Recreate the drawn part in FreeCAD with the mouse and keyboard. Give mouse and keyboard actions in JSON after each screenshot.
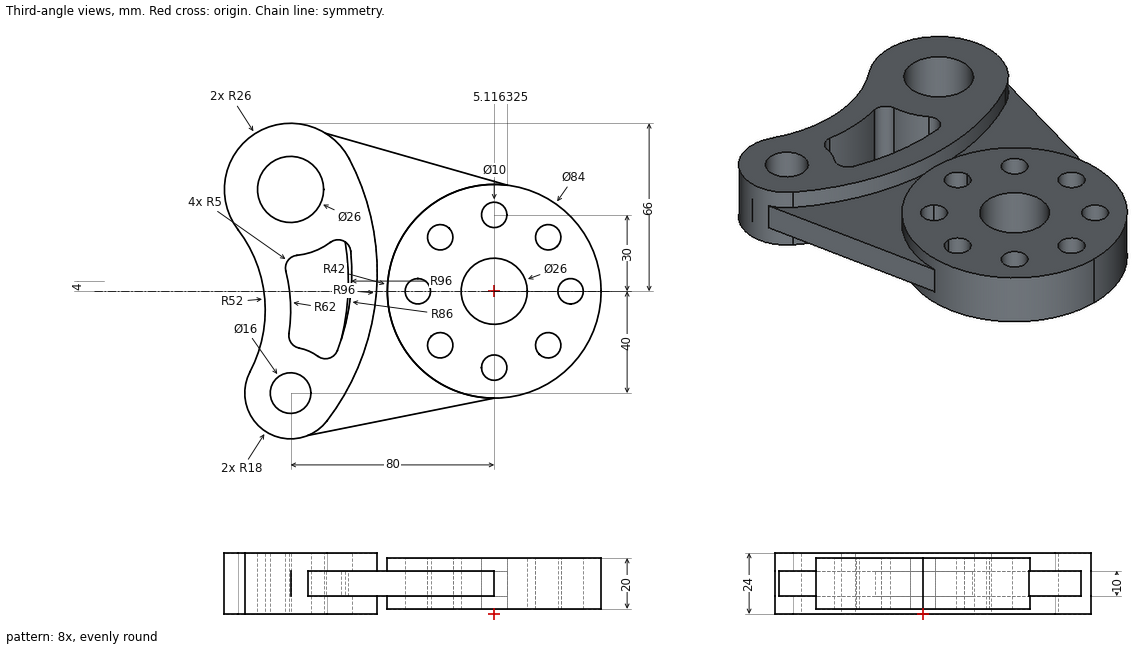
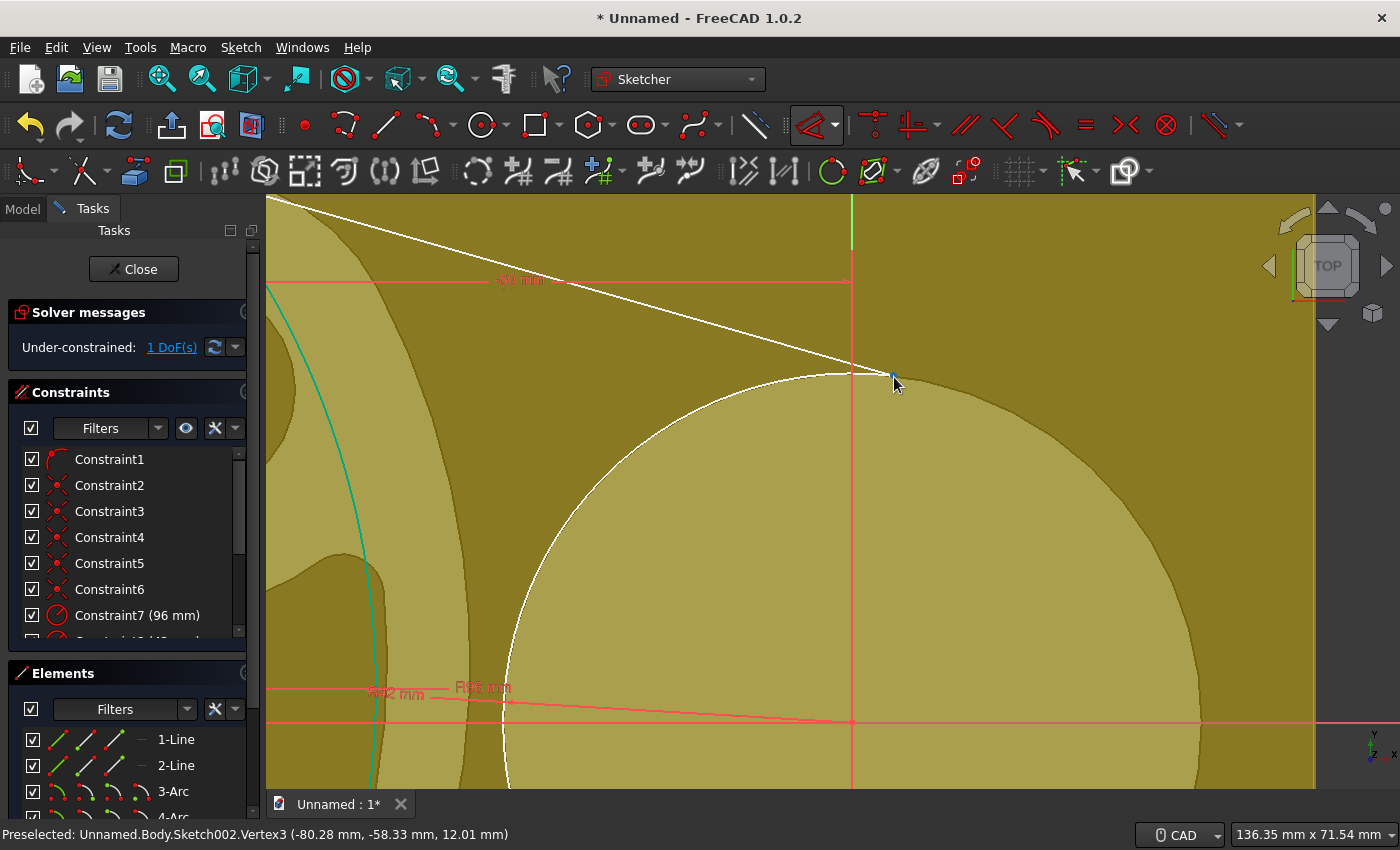
{"action": "left_click", "coordinate": [894, 376]}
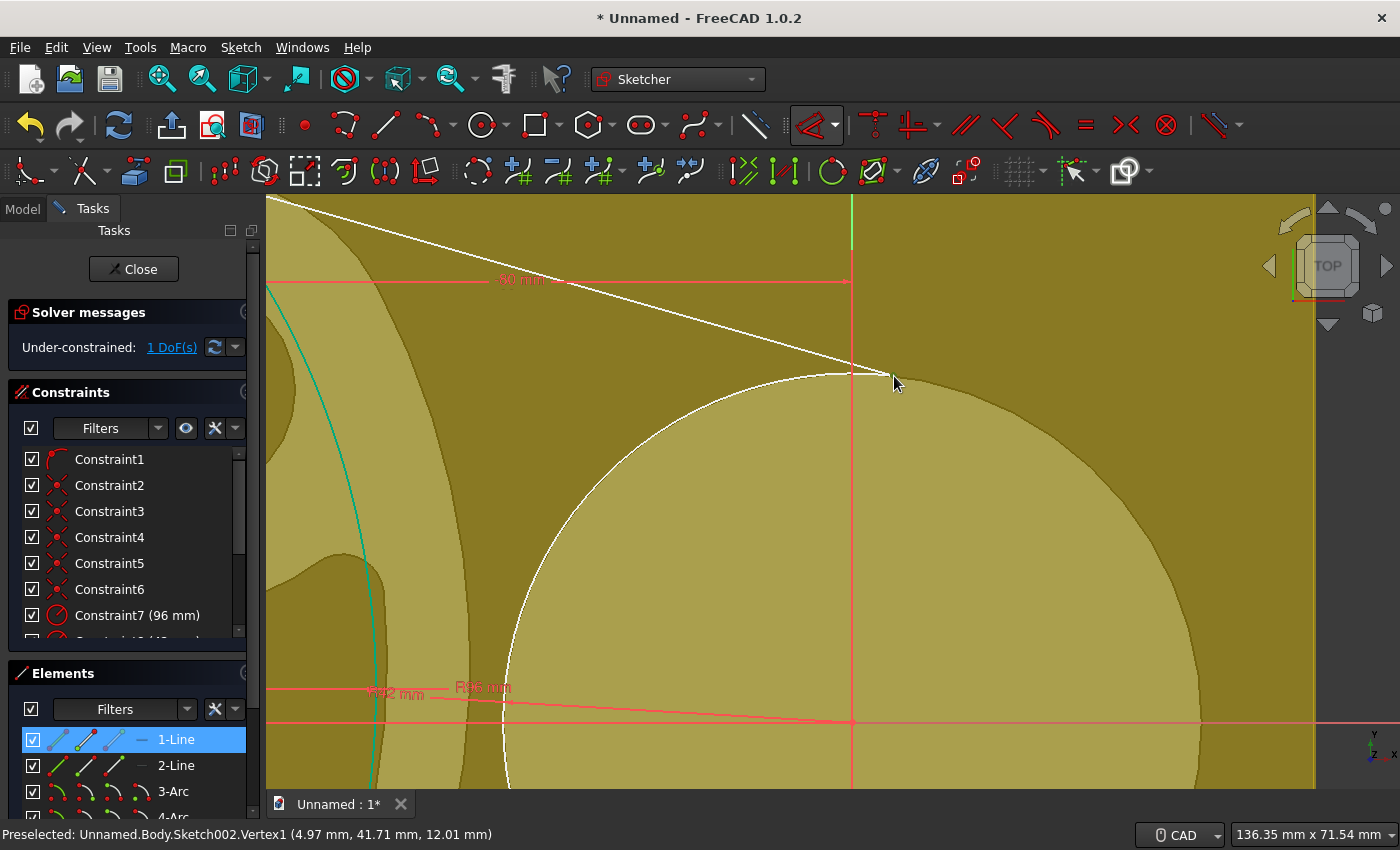
{"action": "left_click", "coordinate": [838, 126]}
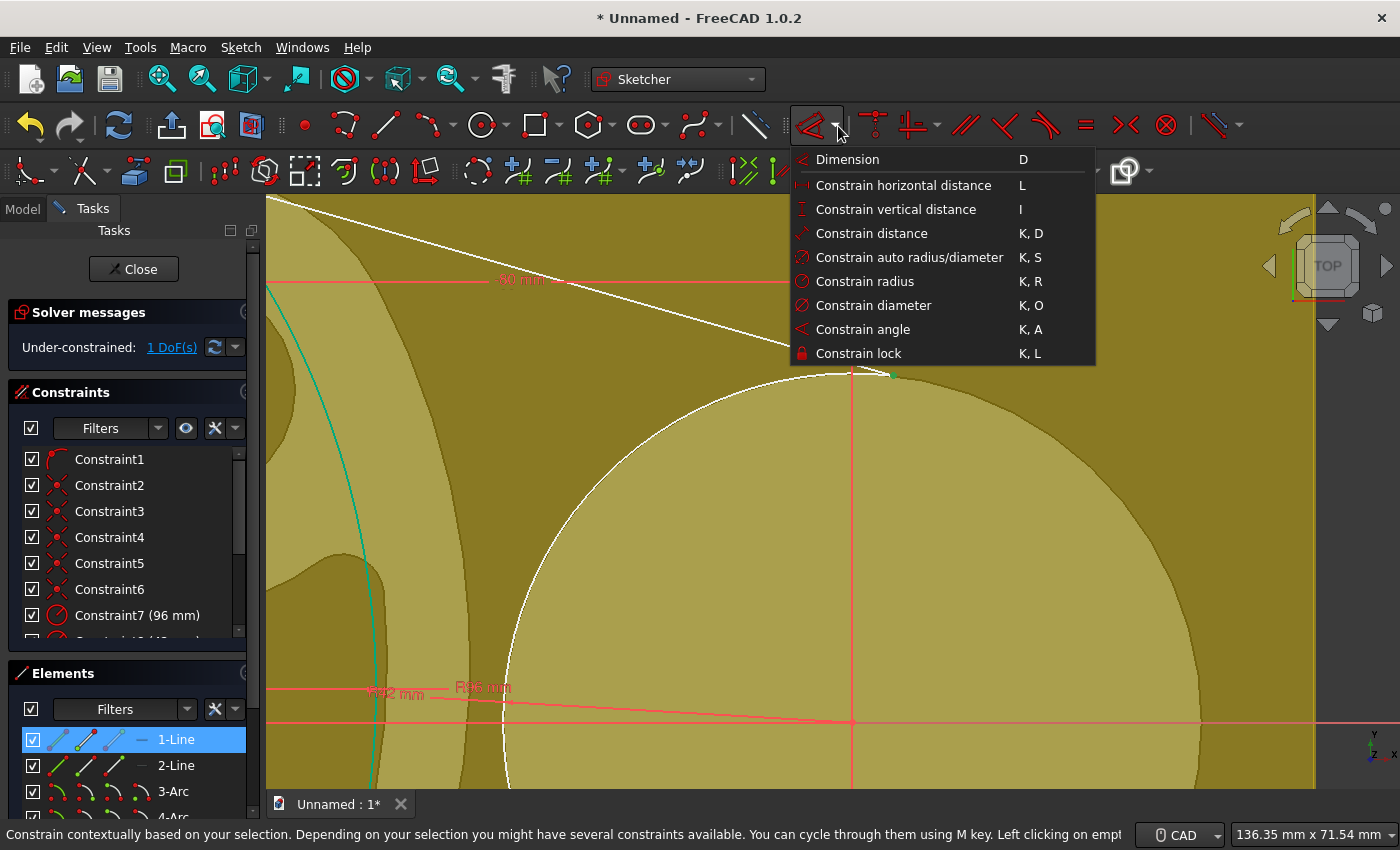
{"action": "left_click", "coordinate": [943, 185]}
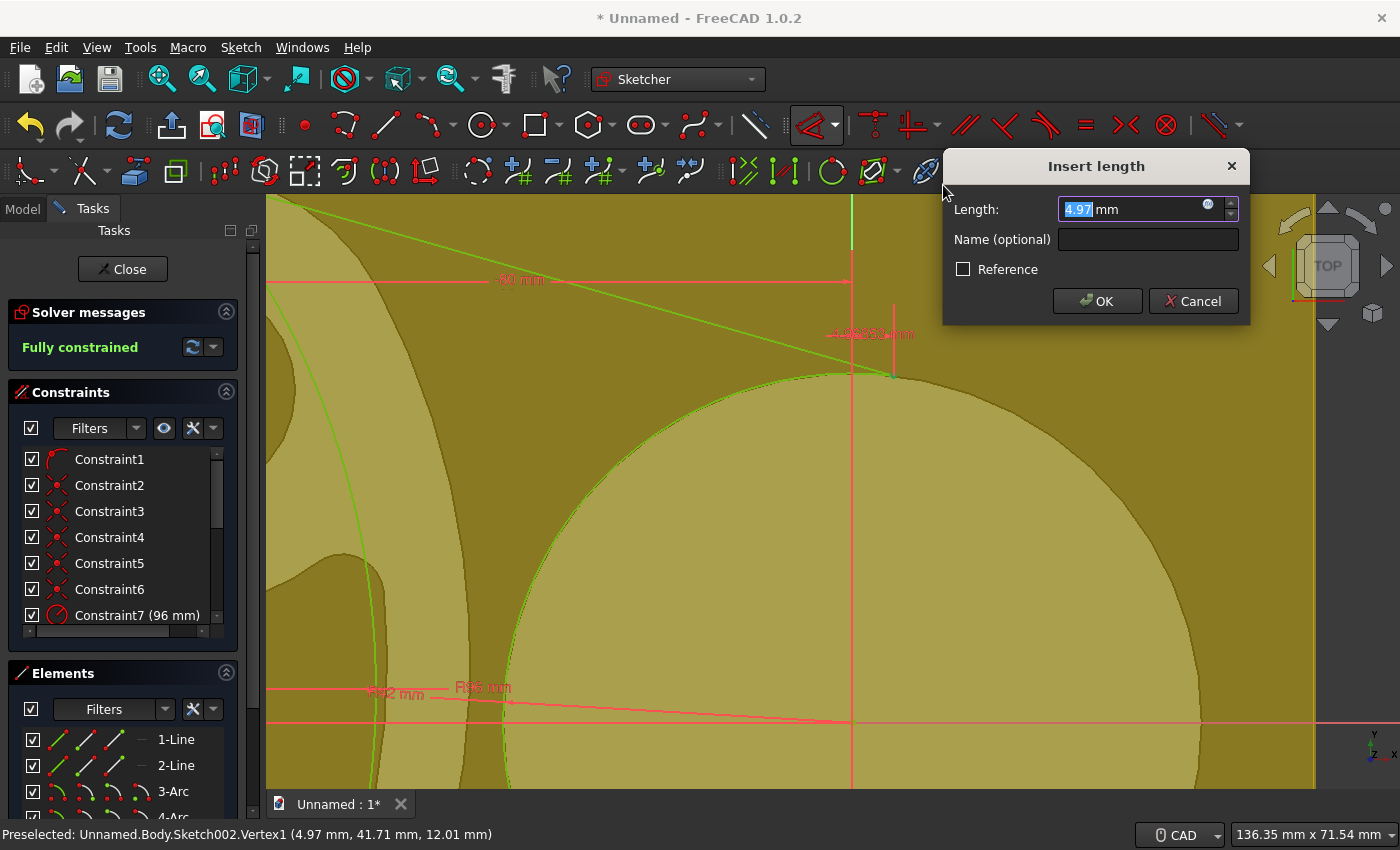
{"action": "type", "text": "5.116325"}
{"action": "key", "text": "Return"}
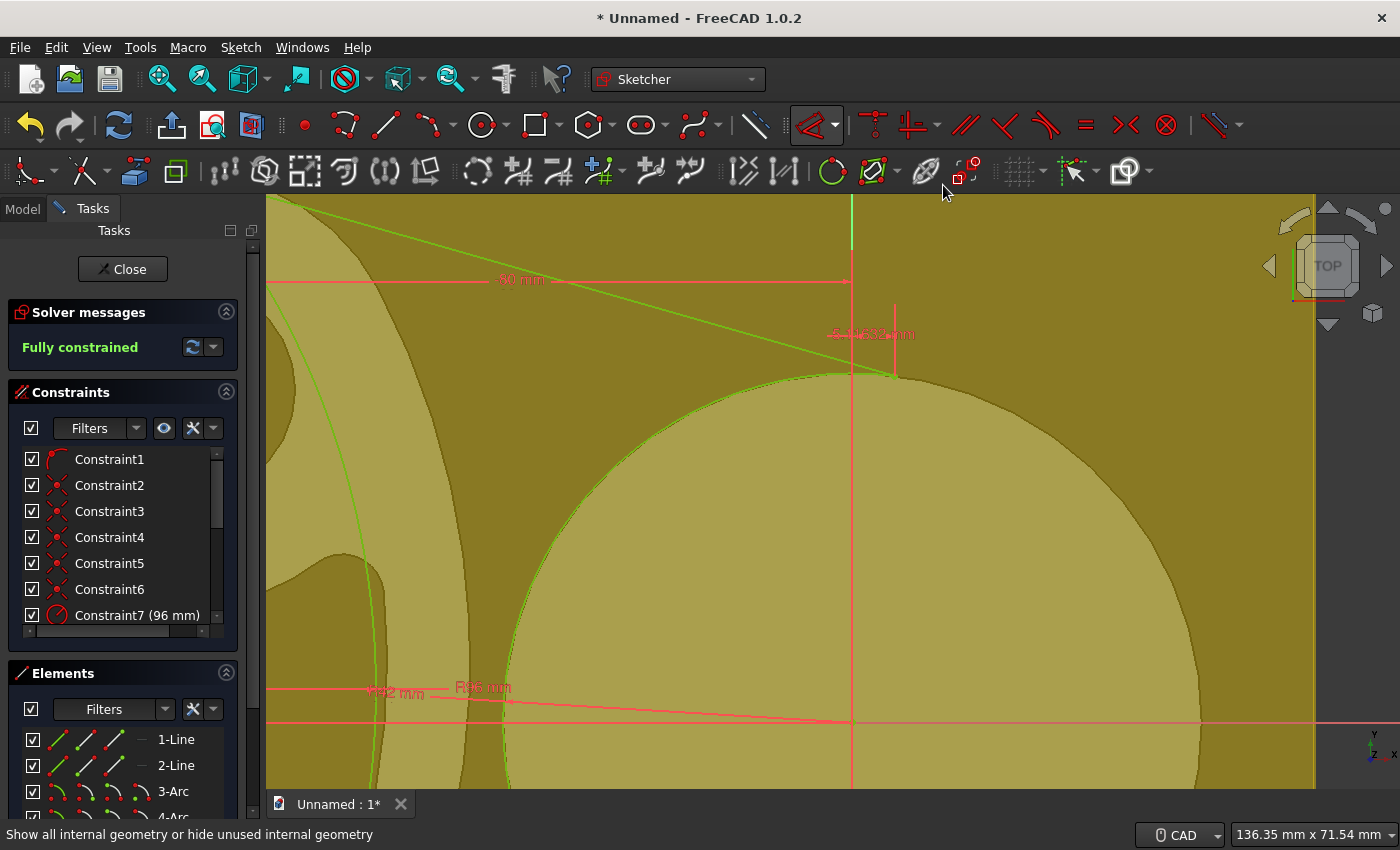
{"action": "left_click", "coordinate": [123, 269]}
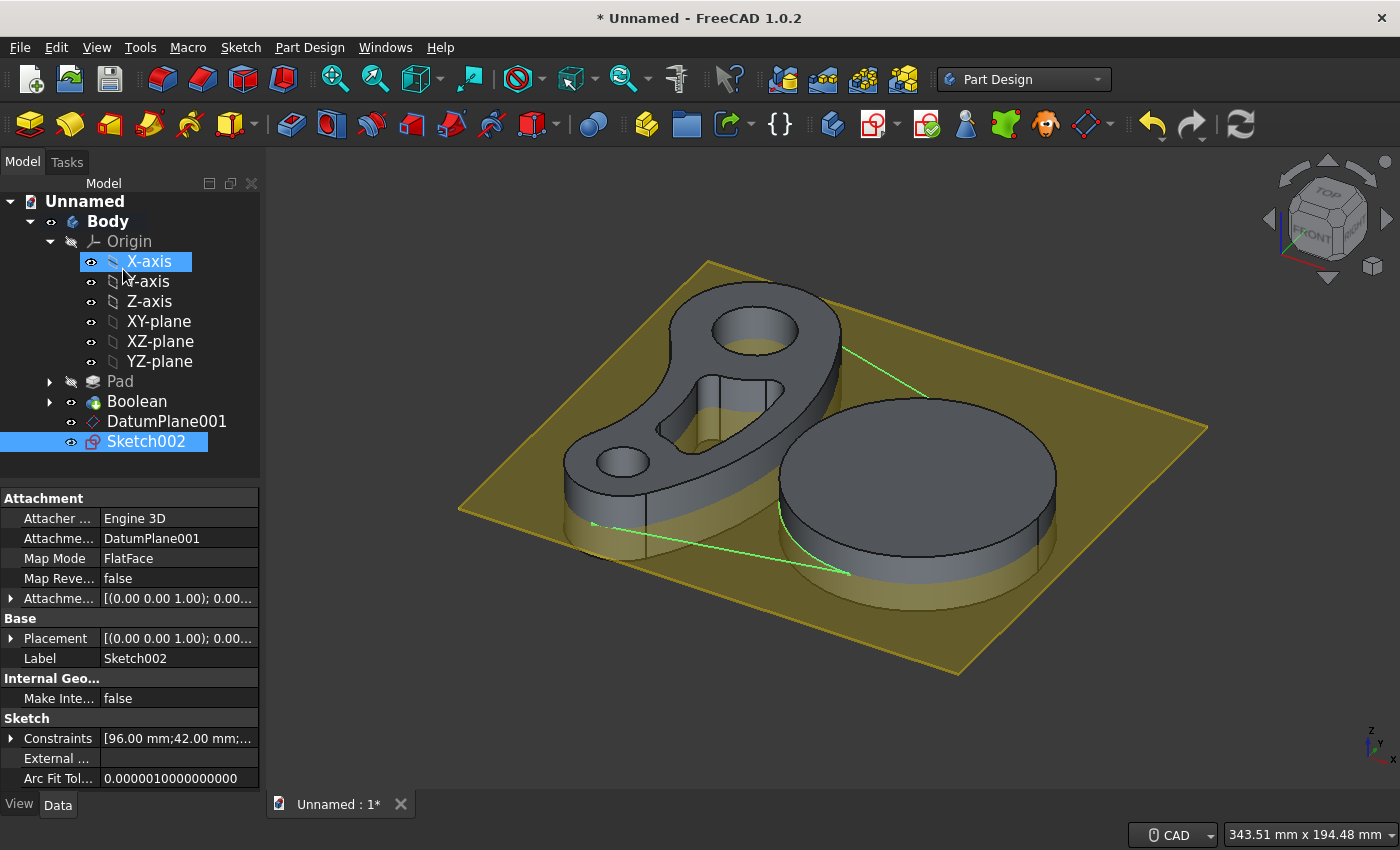
{"action": "left_click", "coordinate": [30, 124]}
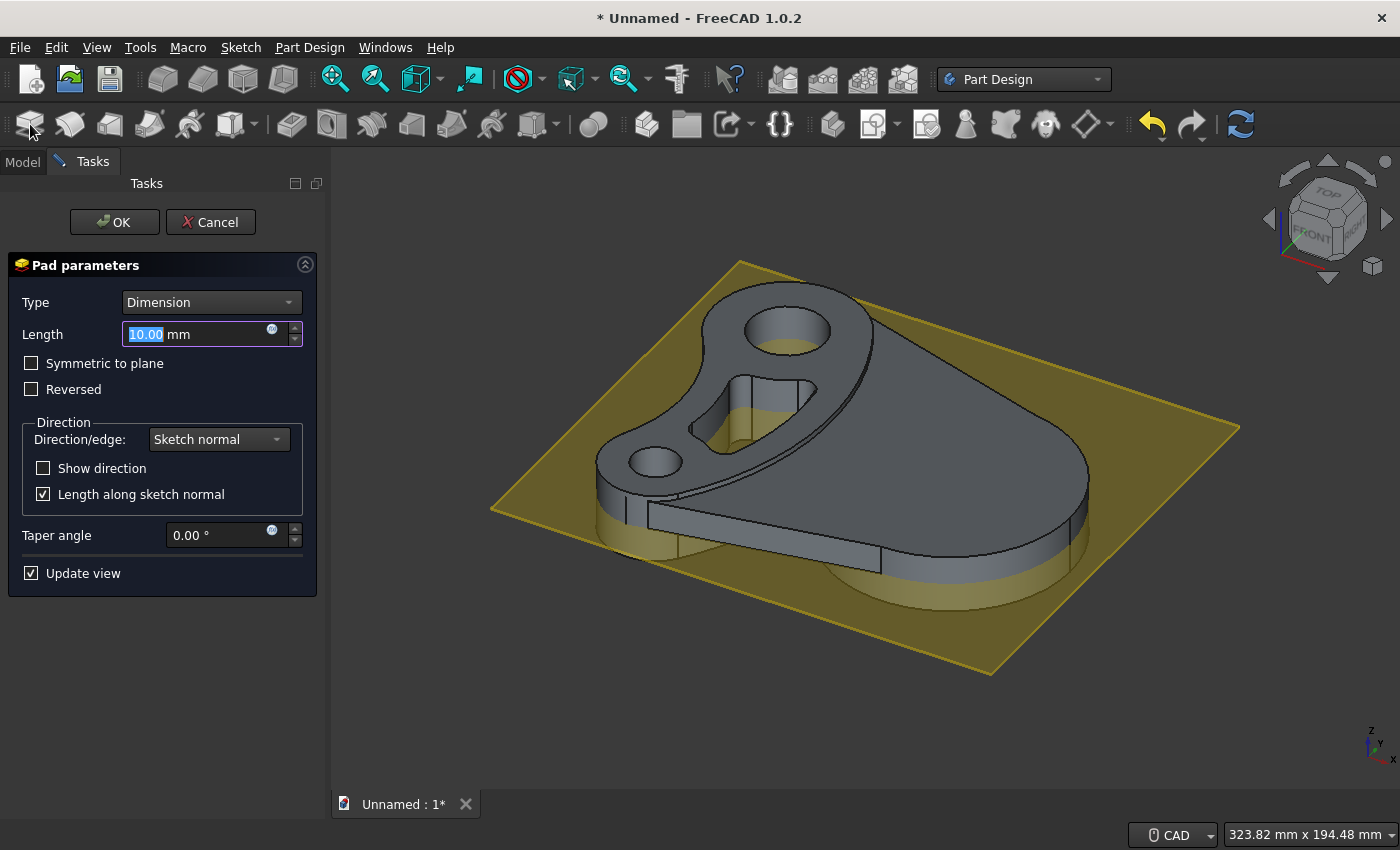
{"action": "type", "text": "10"}
{"action": "key", "text": "Tab"}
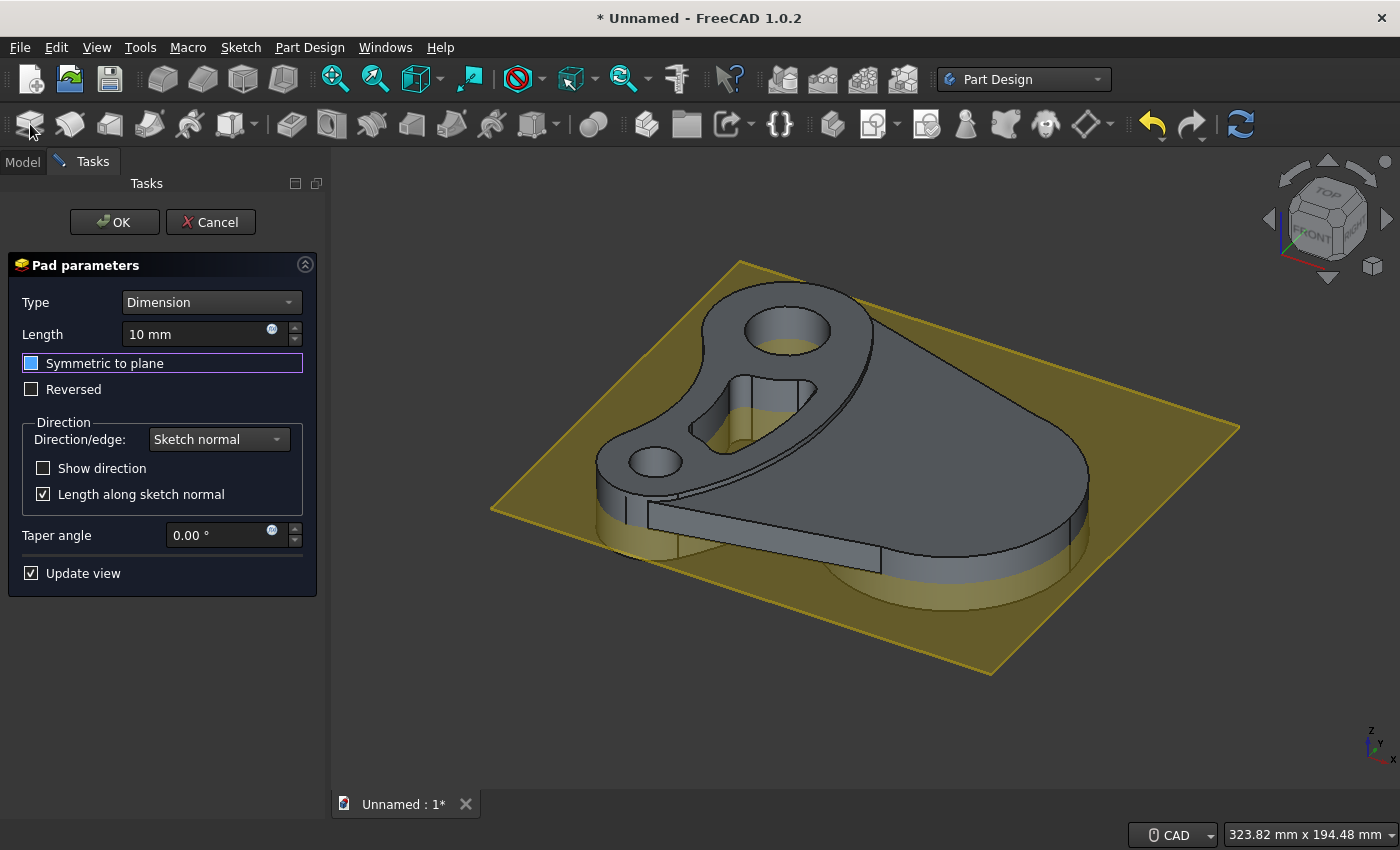
{"action": "left_click", "coordinate": [30, 363]}